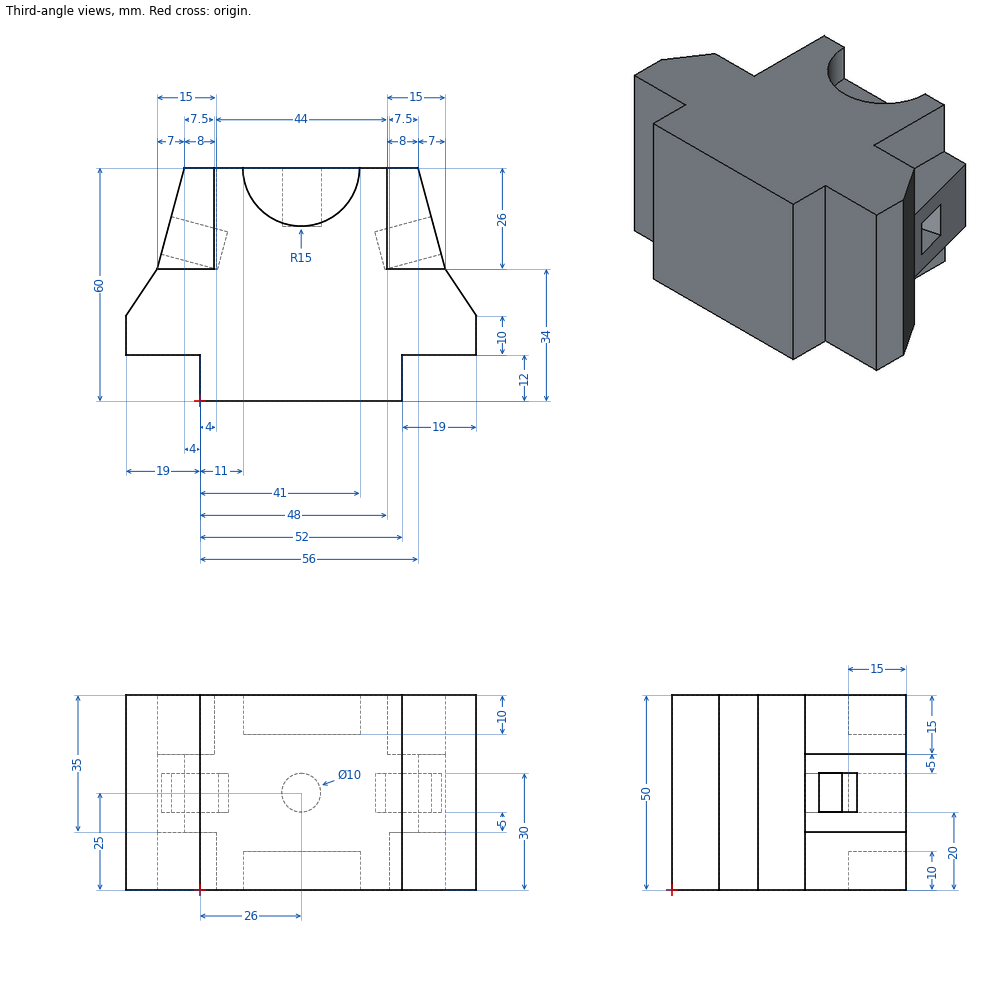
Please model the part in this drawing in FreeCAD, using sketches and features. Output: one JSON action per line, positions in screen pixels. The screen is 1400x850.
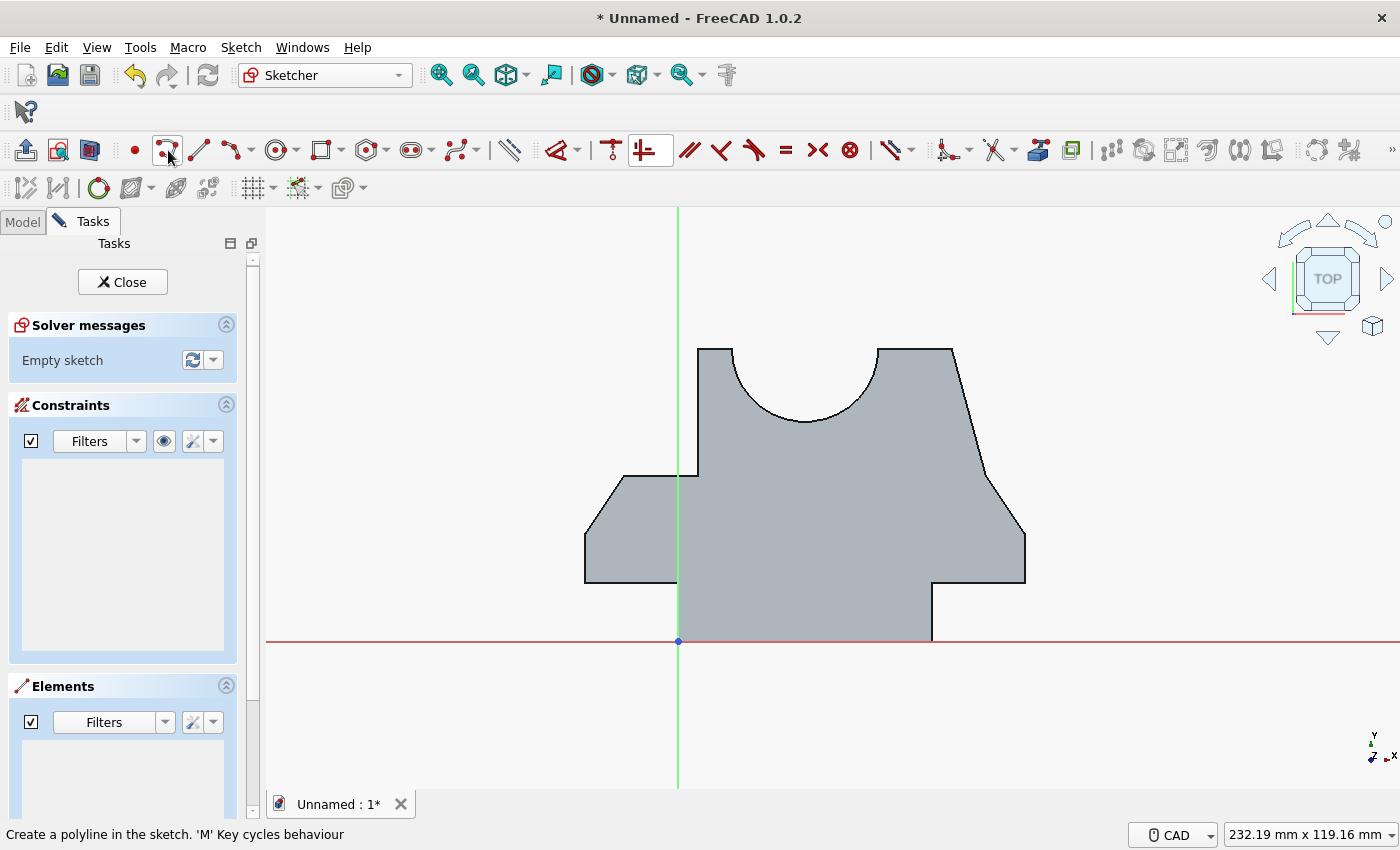
{"action": "left_click", "coordinate": [915, 476]}
{"action": "left_click", "coordinate": [915, 349]}
{"action": "left_click", "coordinate": [952, 349]}
{"action": "left_click", "coordinate": [986, 476]}
{"action": "left_click", "coordinate": [915, 477]}
{"action": "key", "text": "Escape"}
{"action": "key", "text": "Escape"}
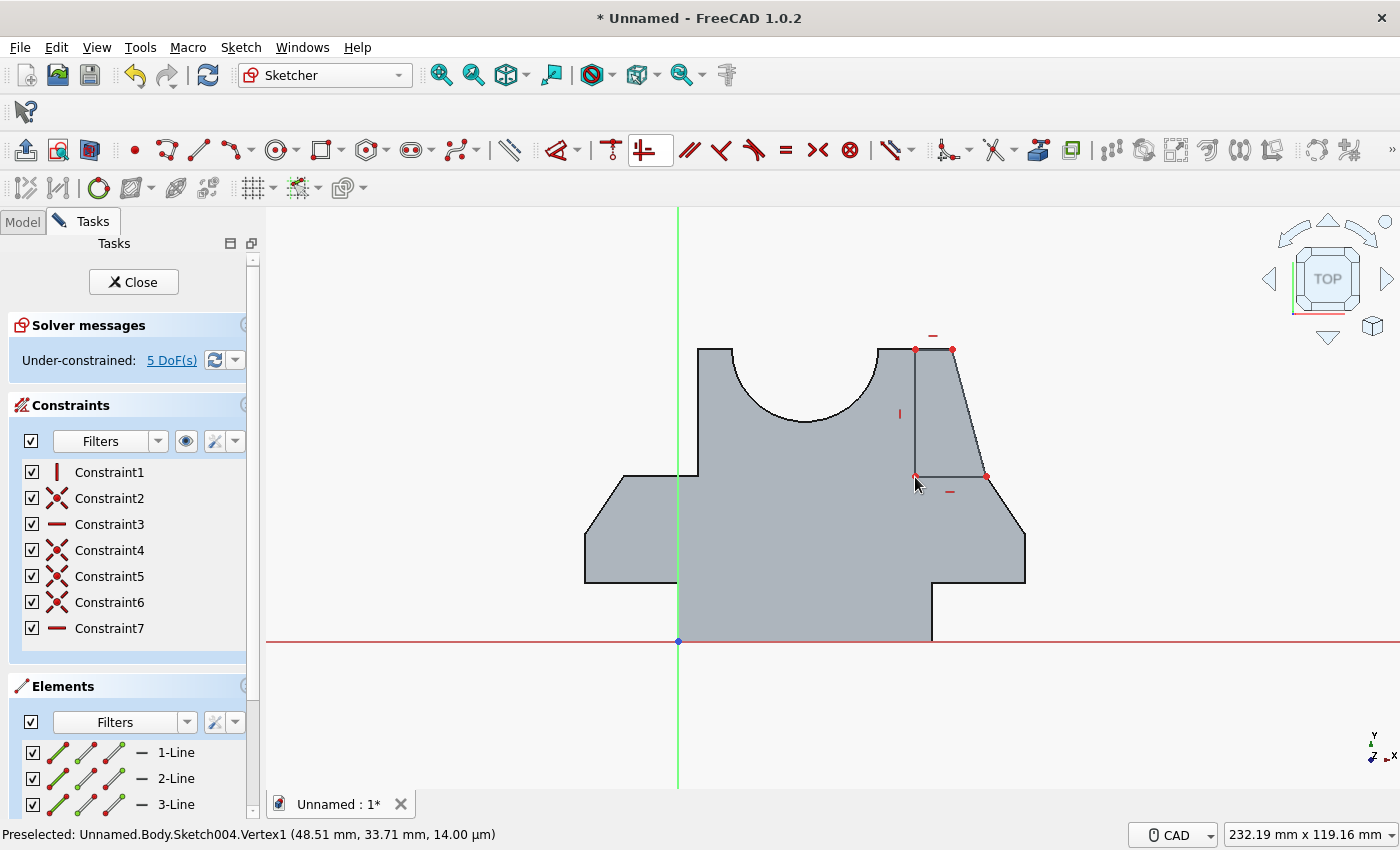
{"action": "left_click", "coordinate": [556, 150]}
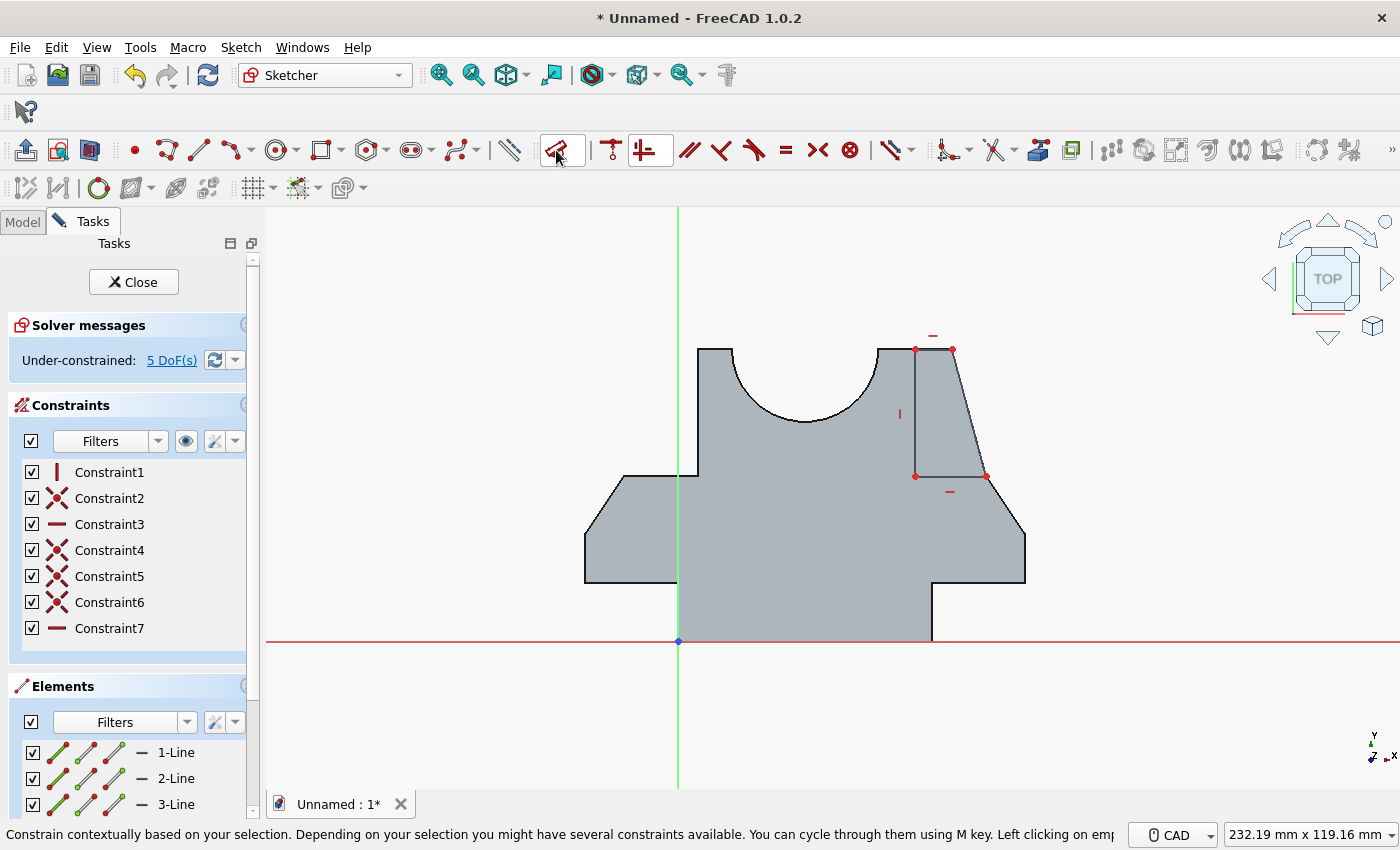
{"action": "left_click", "coordinate": [915, 439]}
{"action": "left_click", "coordinate": [949, 414]}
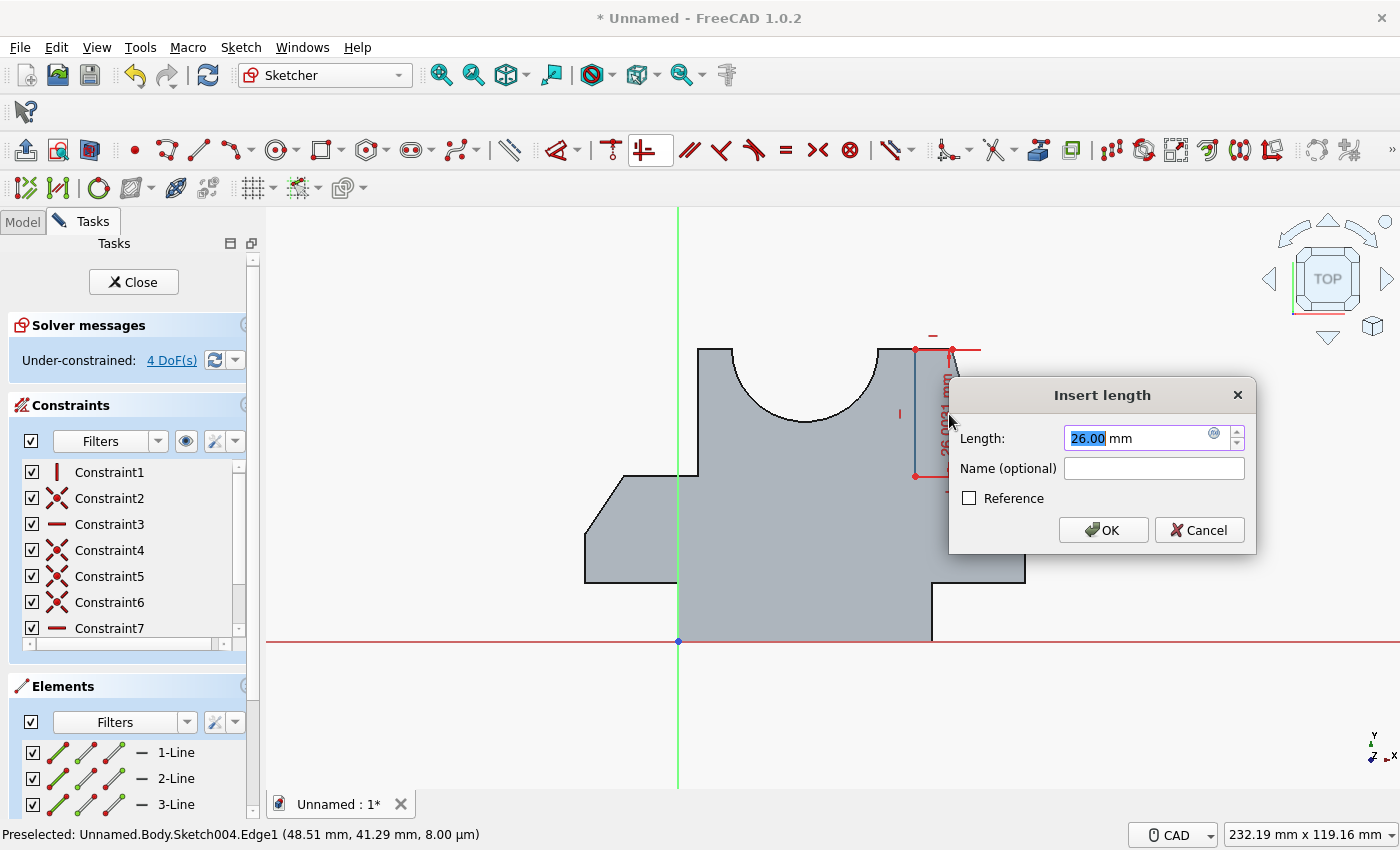
{"action": "type", "text": "26"}
{"action": "key", "text": "Return"}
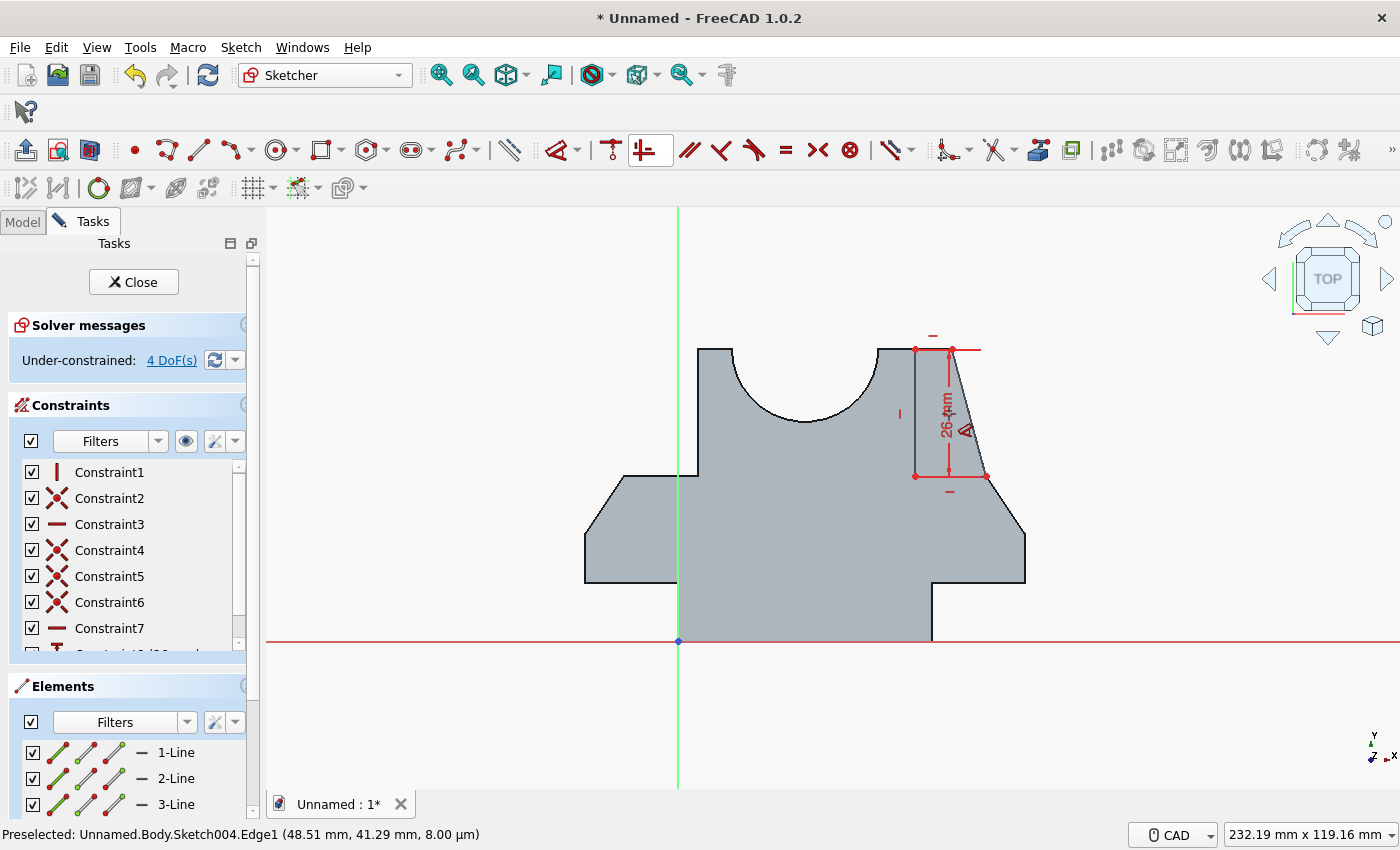
{"action": "left_click", "coordinate": [962, 388]}
{"action": "left_click", "coordinate": [969, 316]}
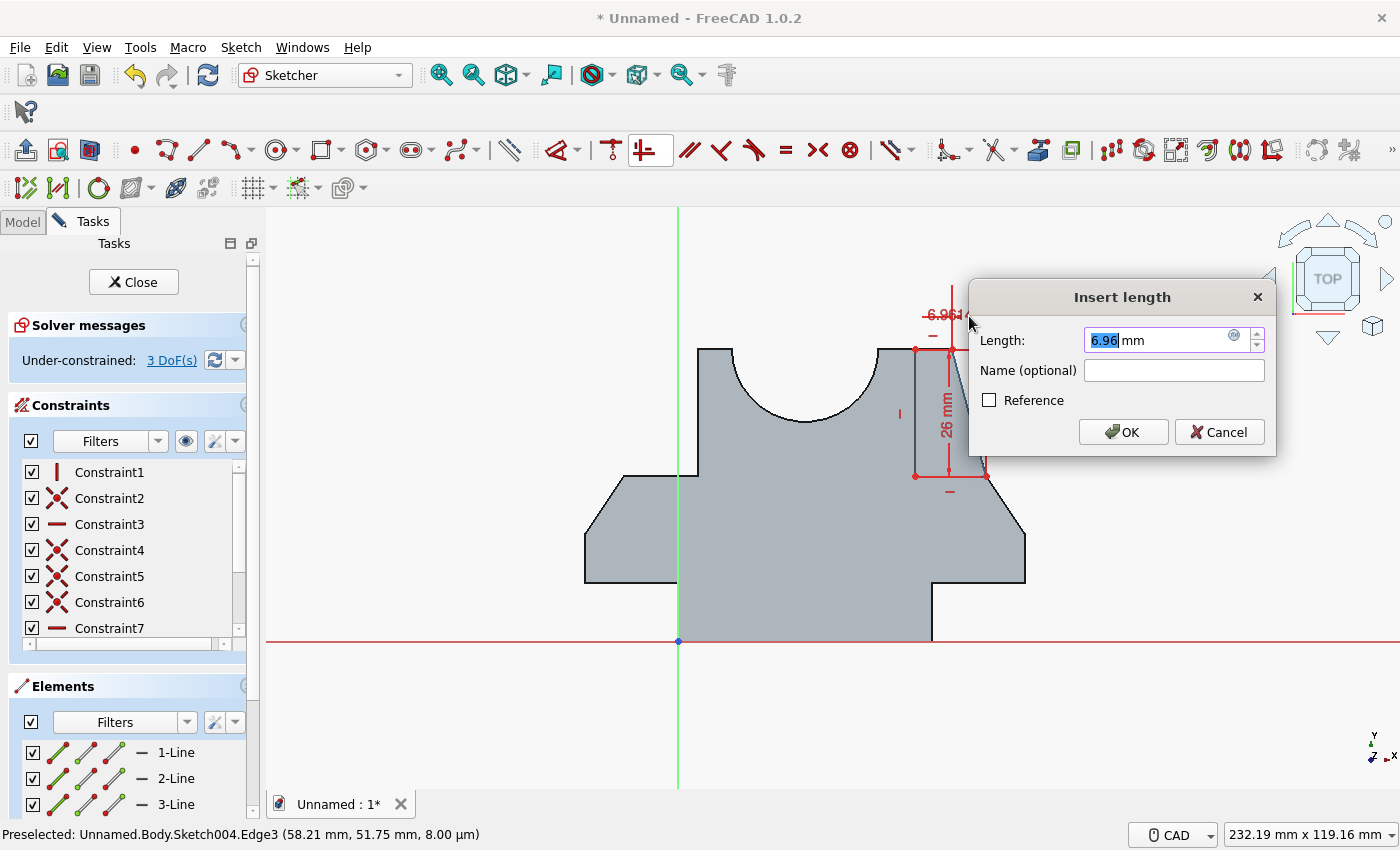
{"action": "type", "text": "7"}
{"action": "key", "text": "Return"}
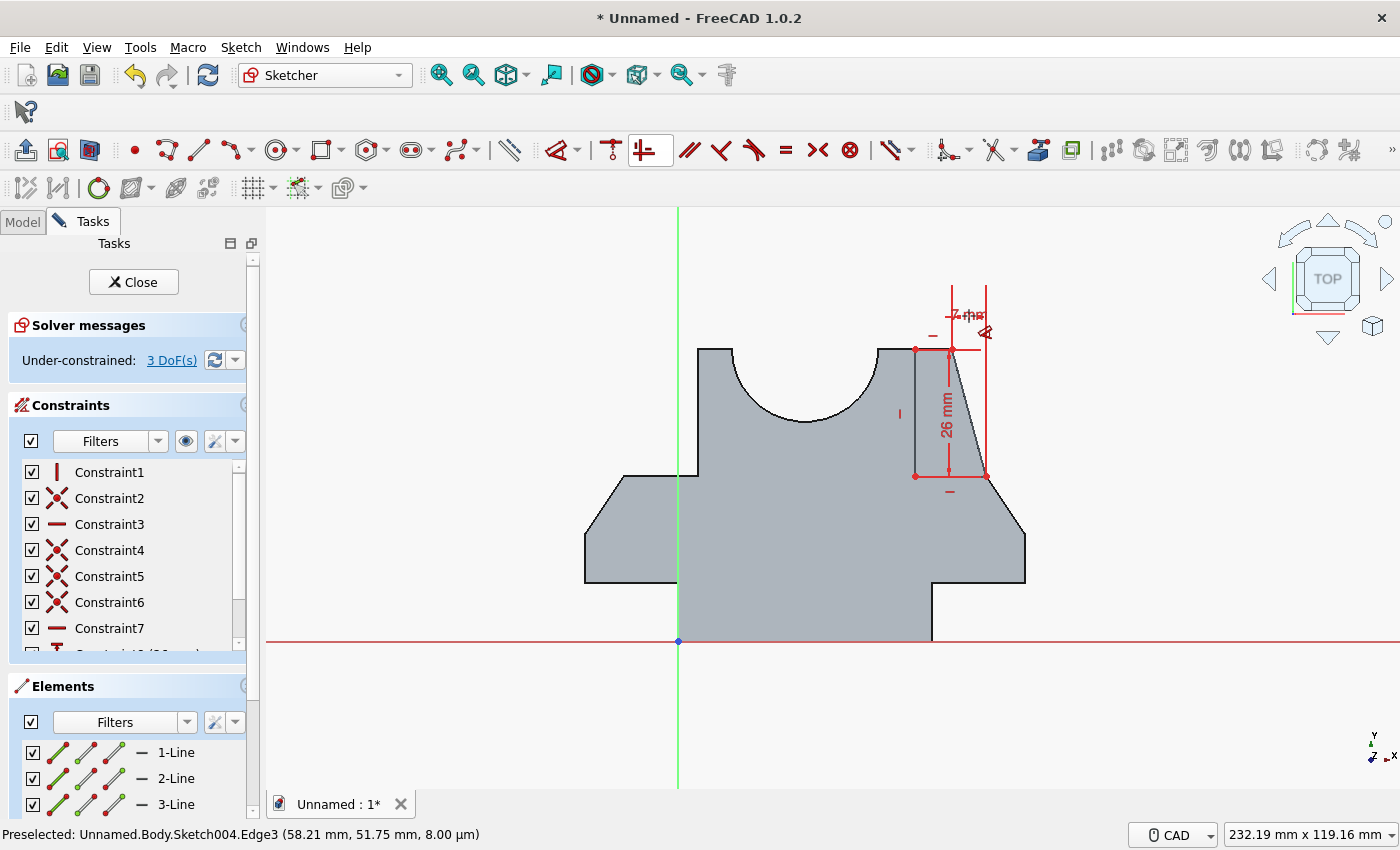
{"action": "scroll", "coordinate": [926, 350], "scroll_direction": "up", "scroll_amount": 2}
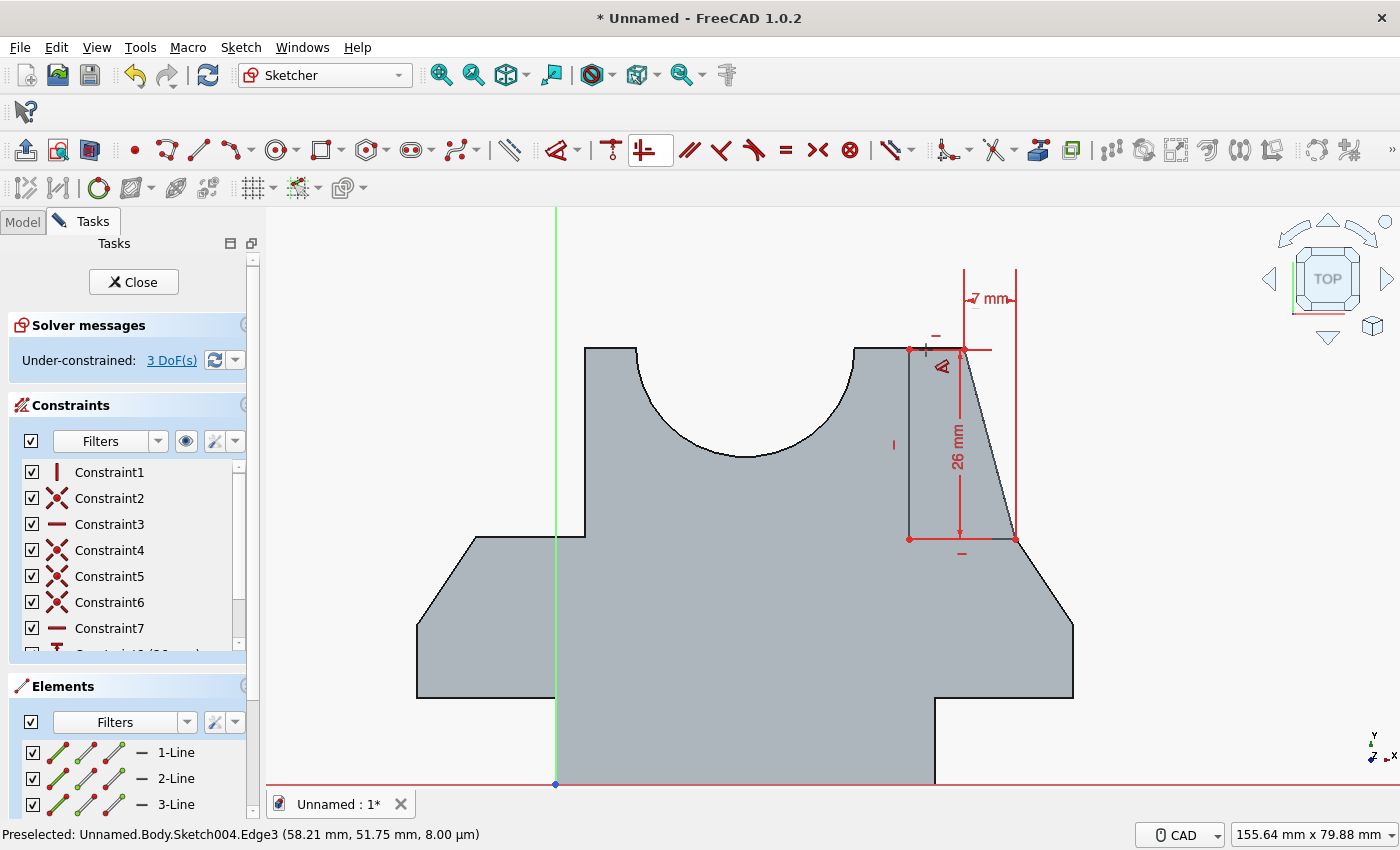
{"action": "left_click", "coordinate": [926, 350]}
{"action": "left_click", "coordinate": [918, 316]}